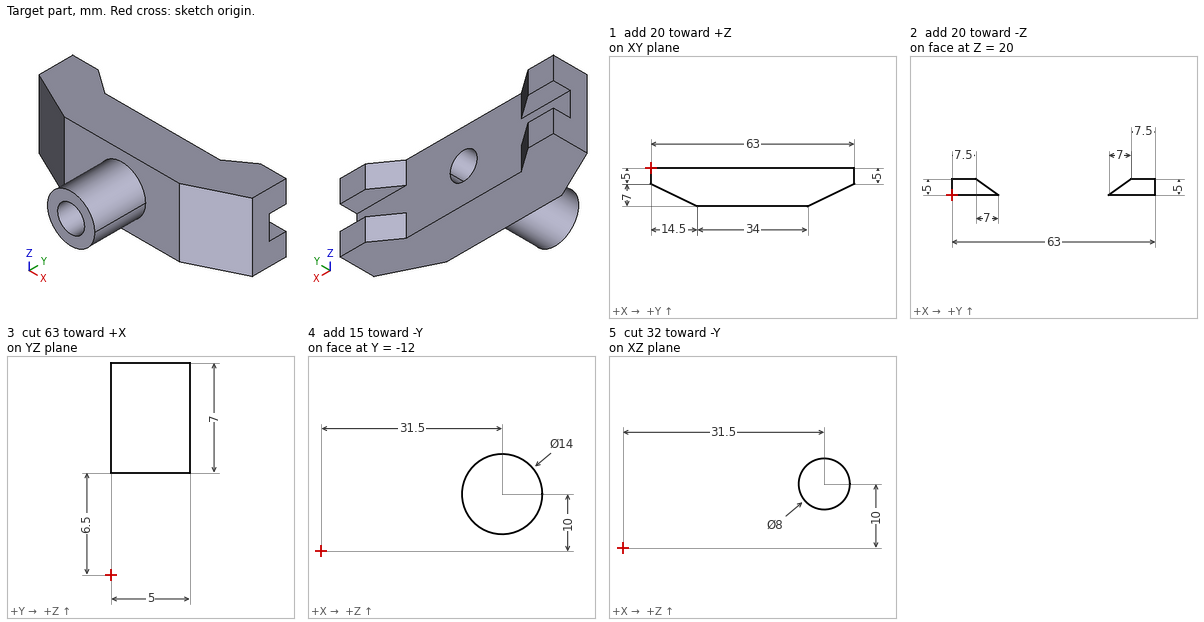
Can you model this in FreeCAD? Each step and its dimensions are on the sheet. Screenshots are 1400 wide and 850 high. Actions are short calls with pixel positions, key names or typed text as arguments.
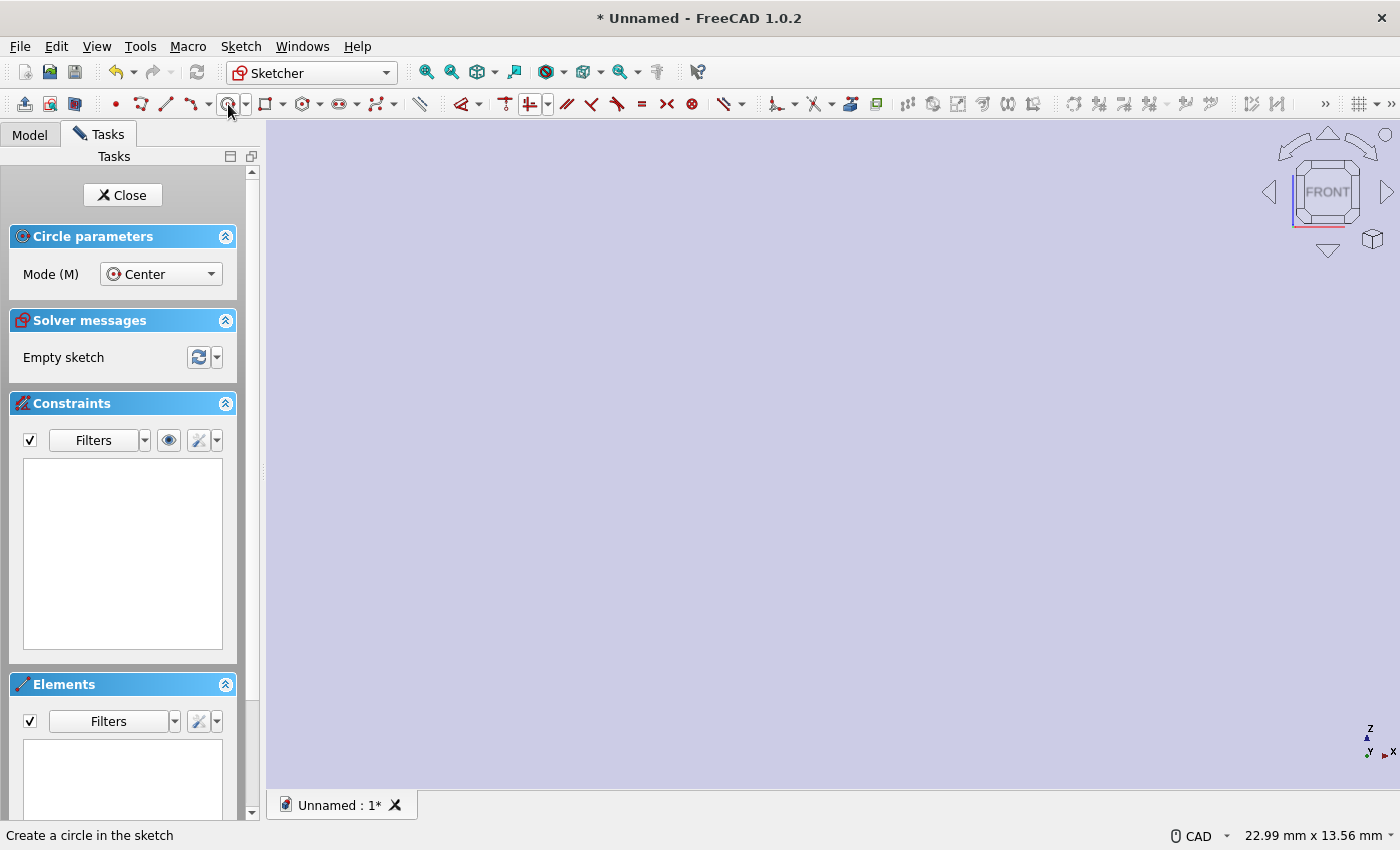
click(764, 454)
move(904, 314)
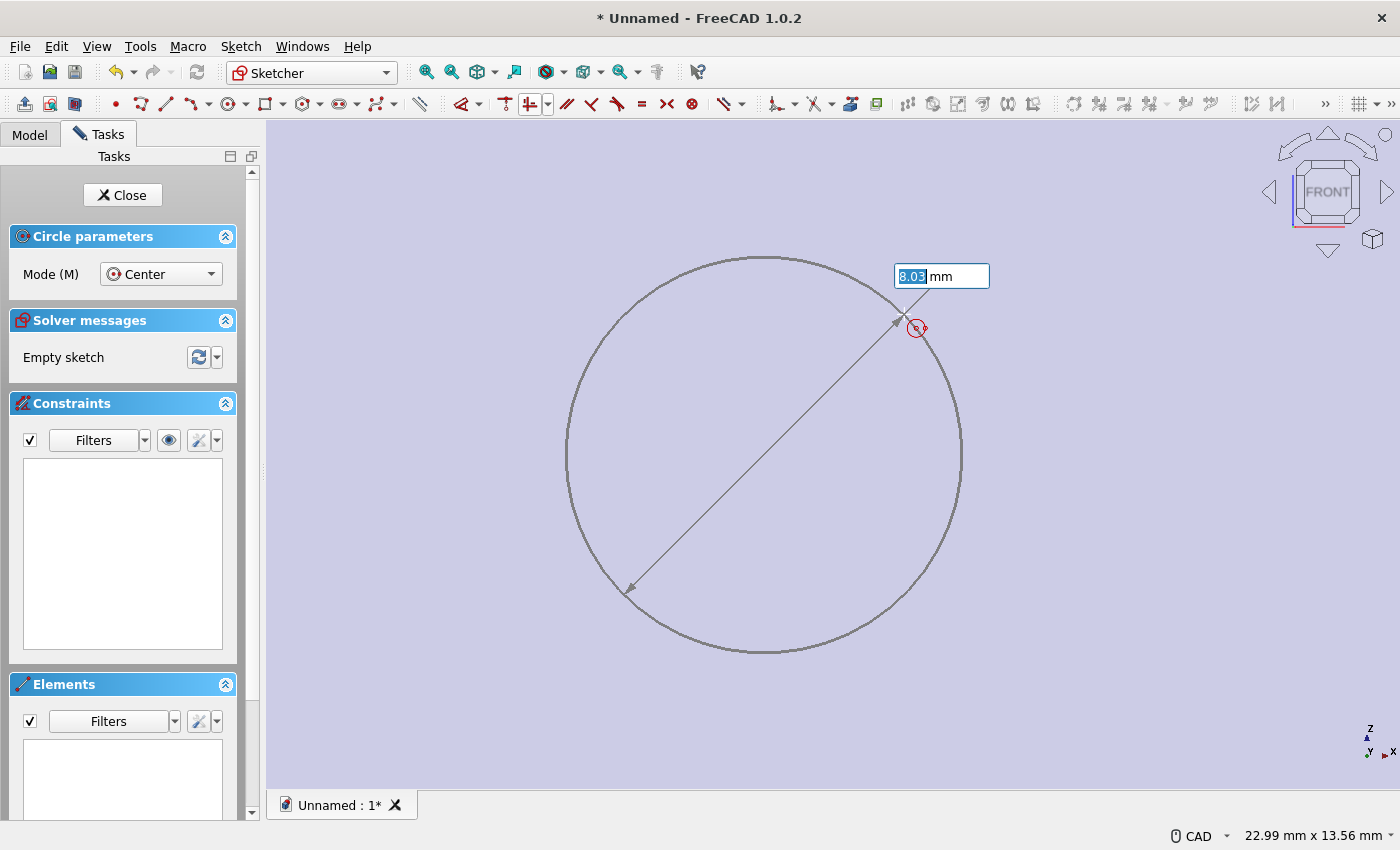
text(8)
key(Return)
key(Escape)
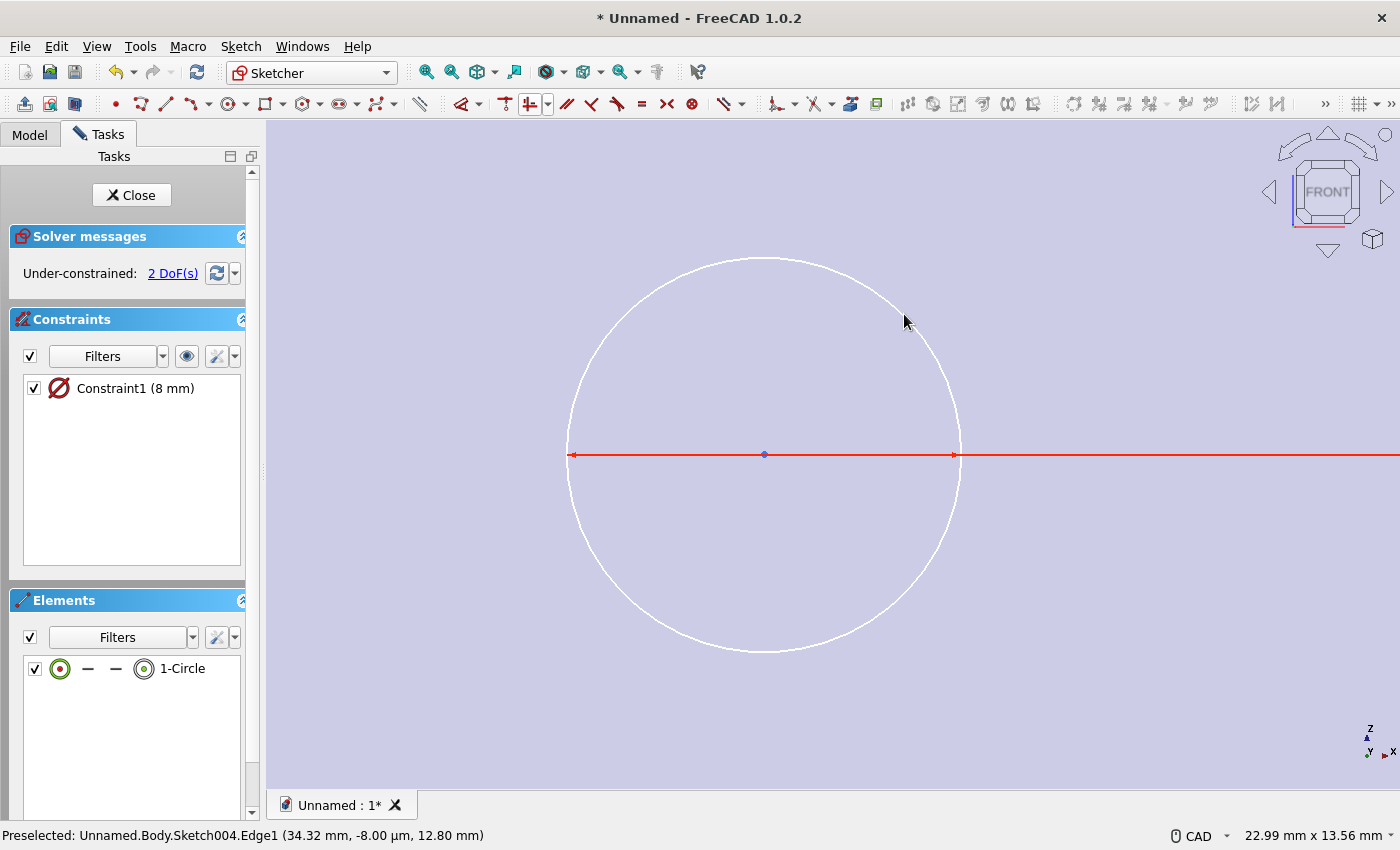
click(460, 104)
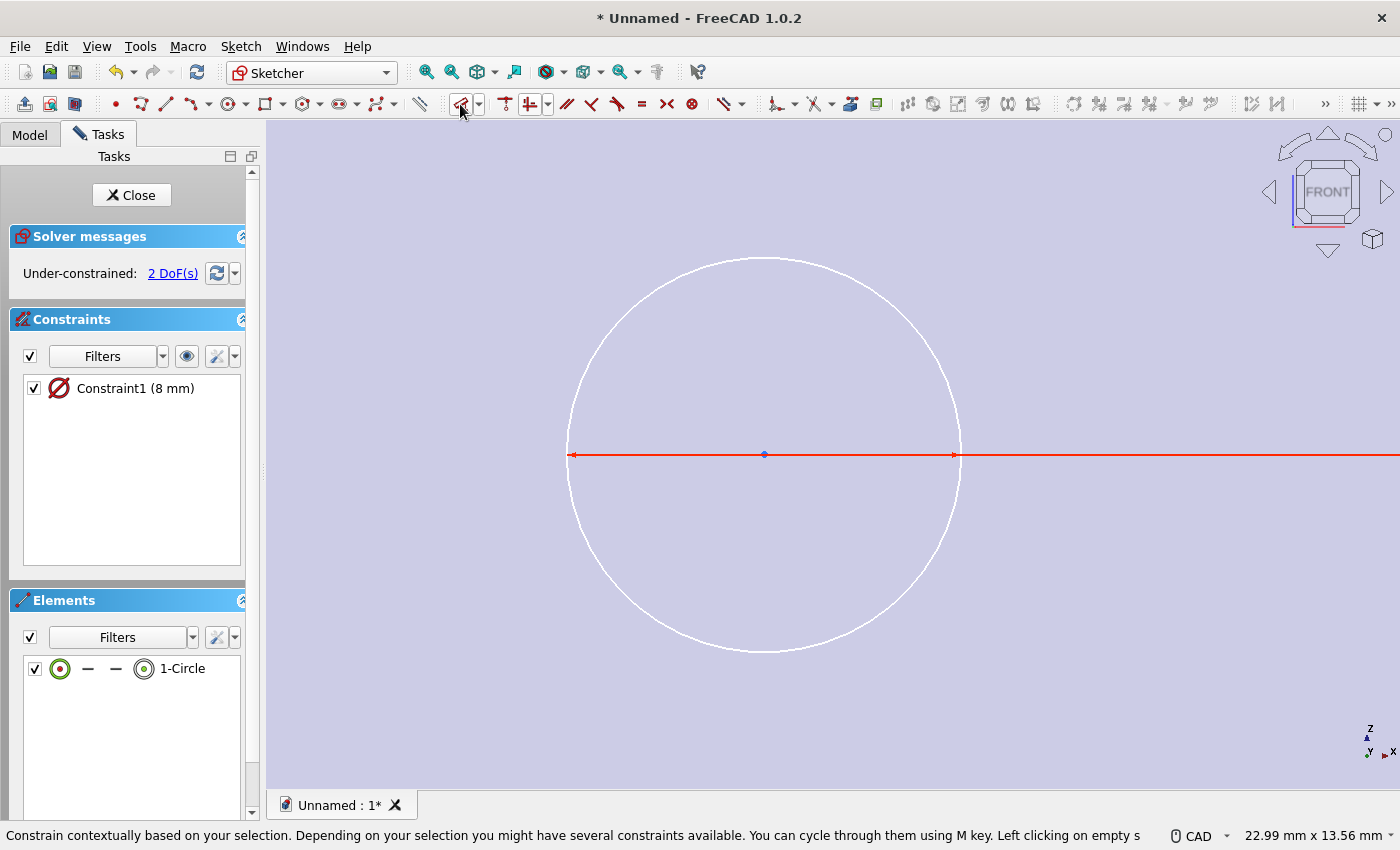
click(764, 455)
click(798, 608)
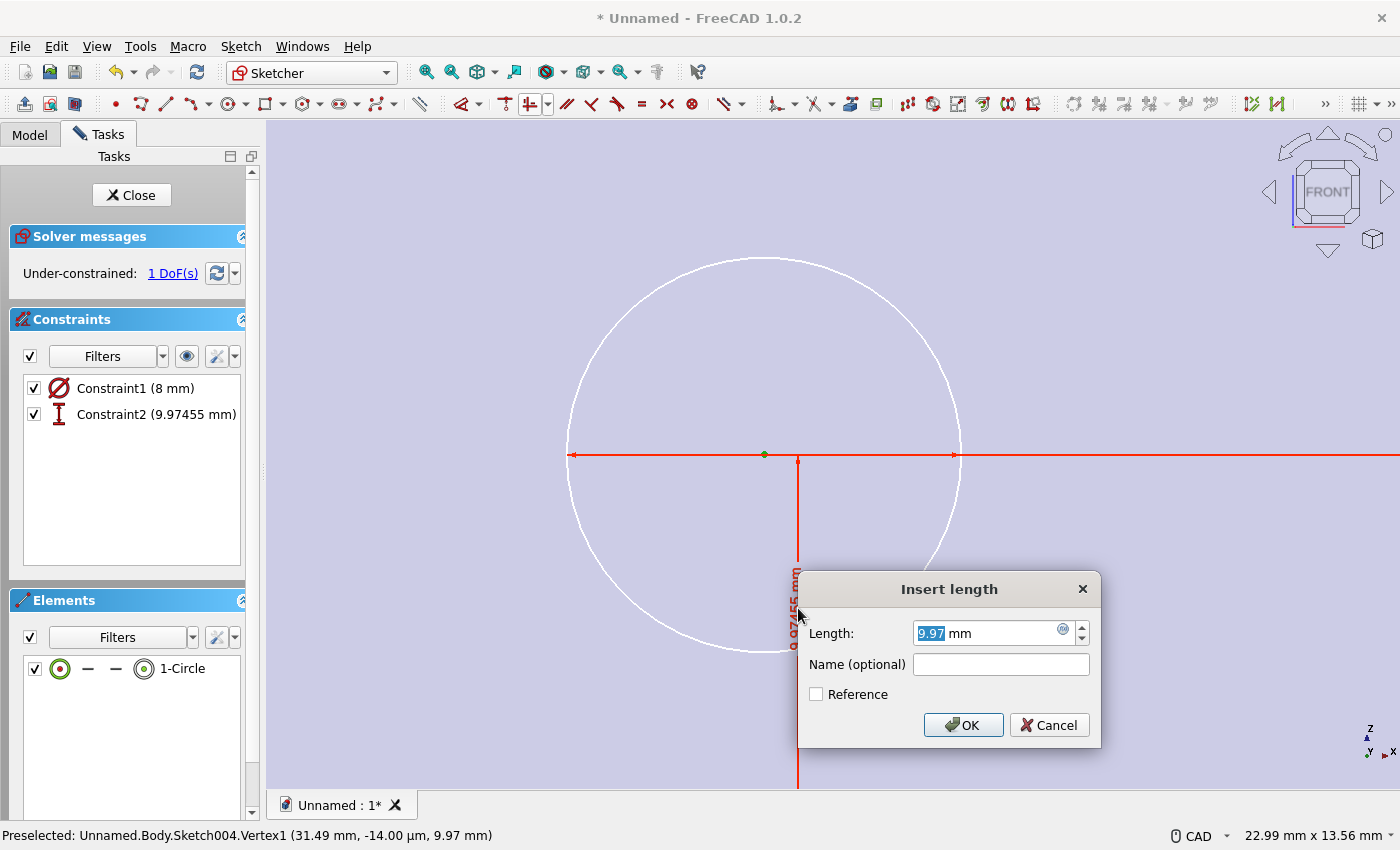
text(10)
key(Return)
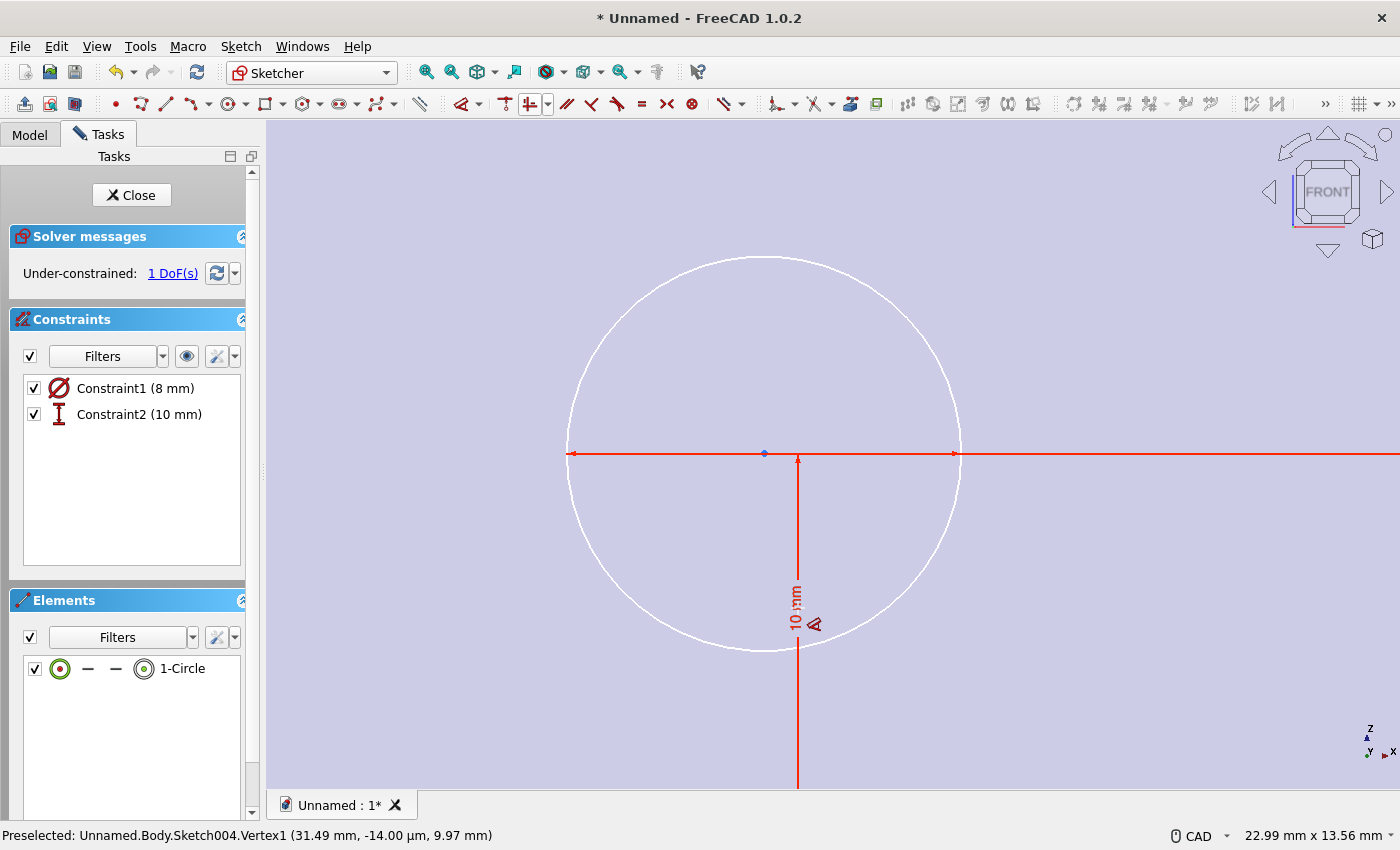
click(764, 454)
click(529, 420)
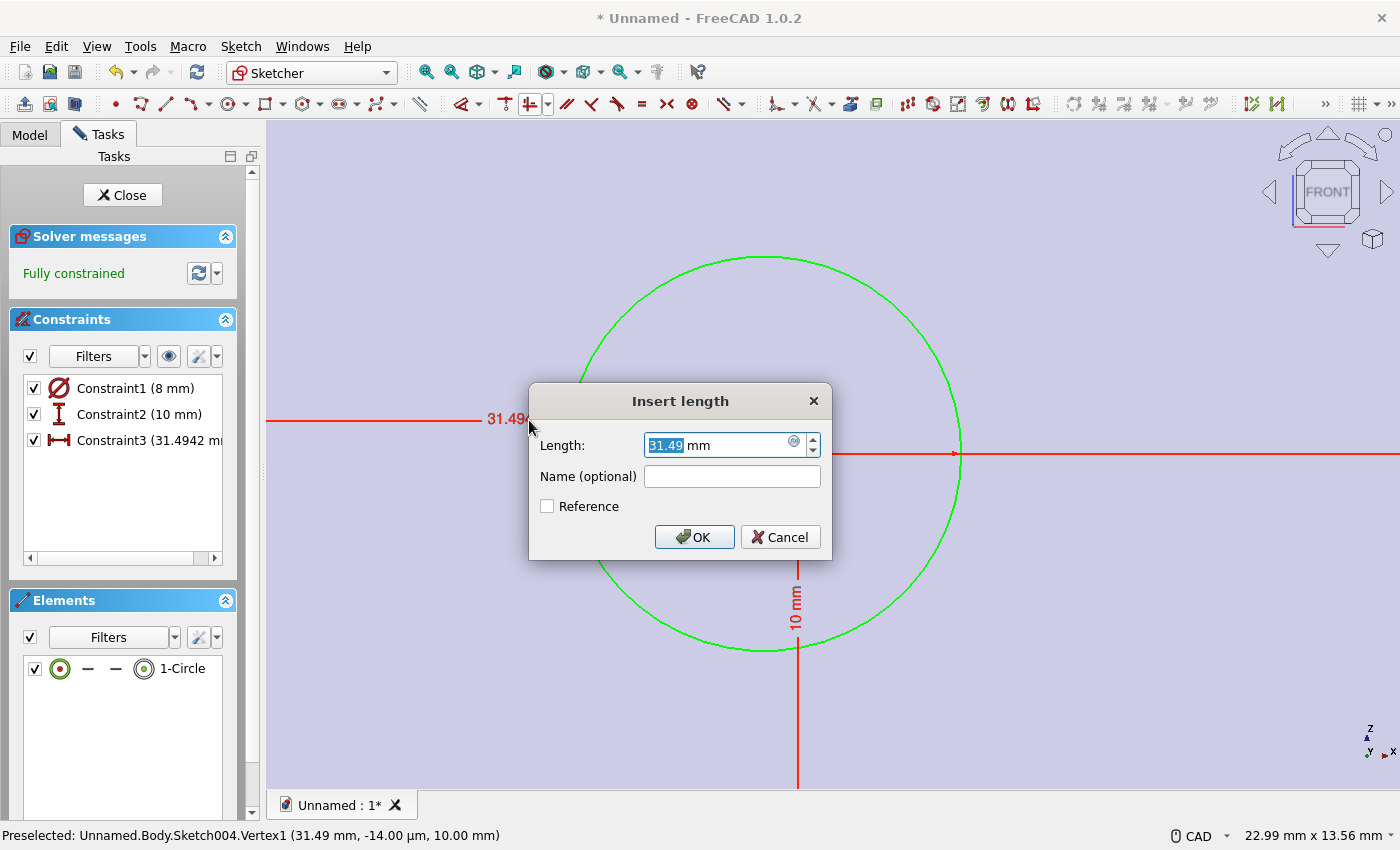
text(31.5)
key(Return)
key(Escape)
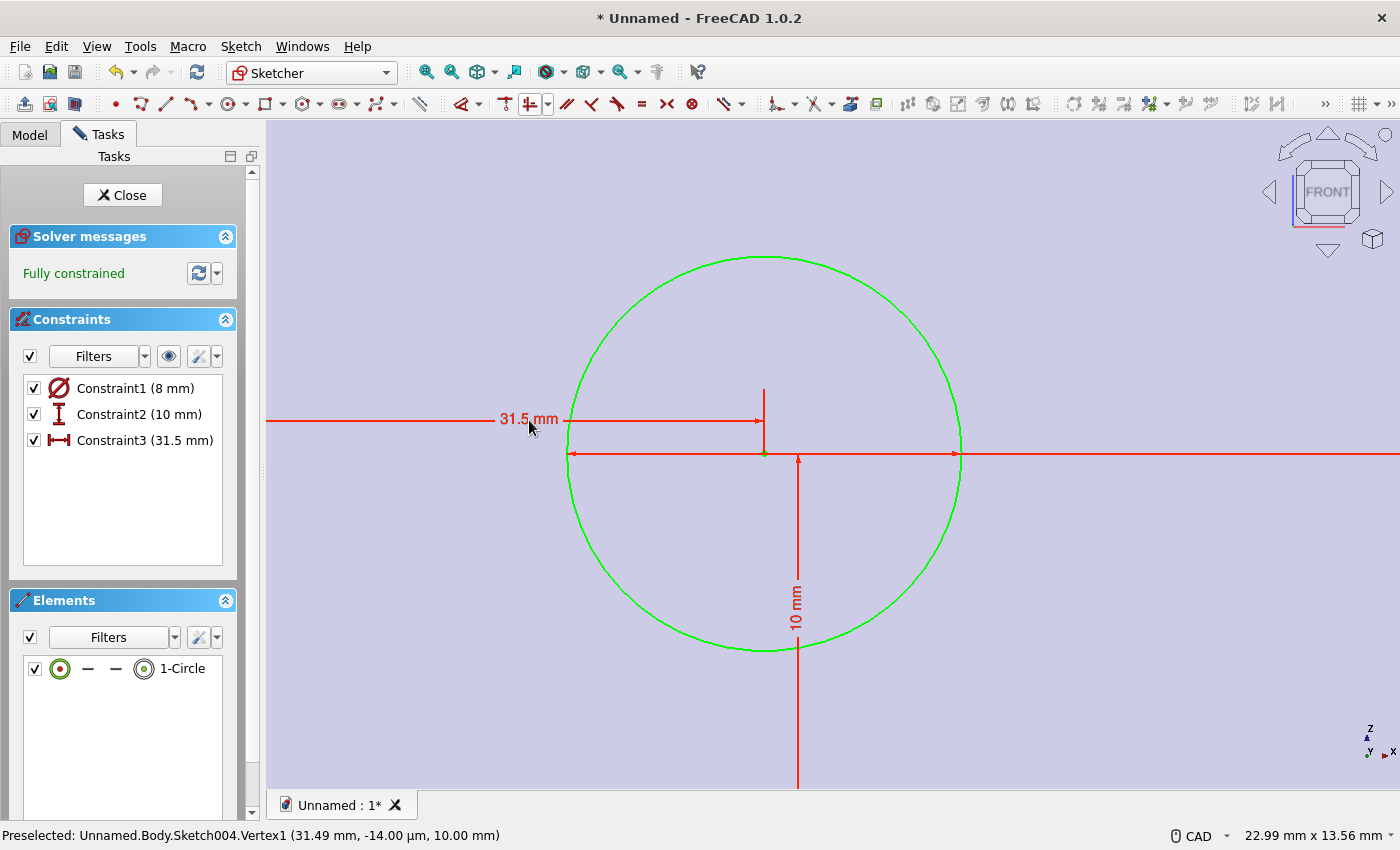
click(123, 195)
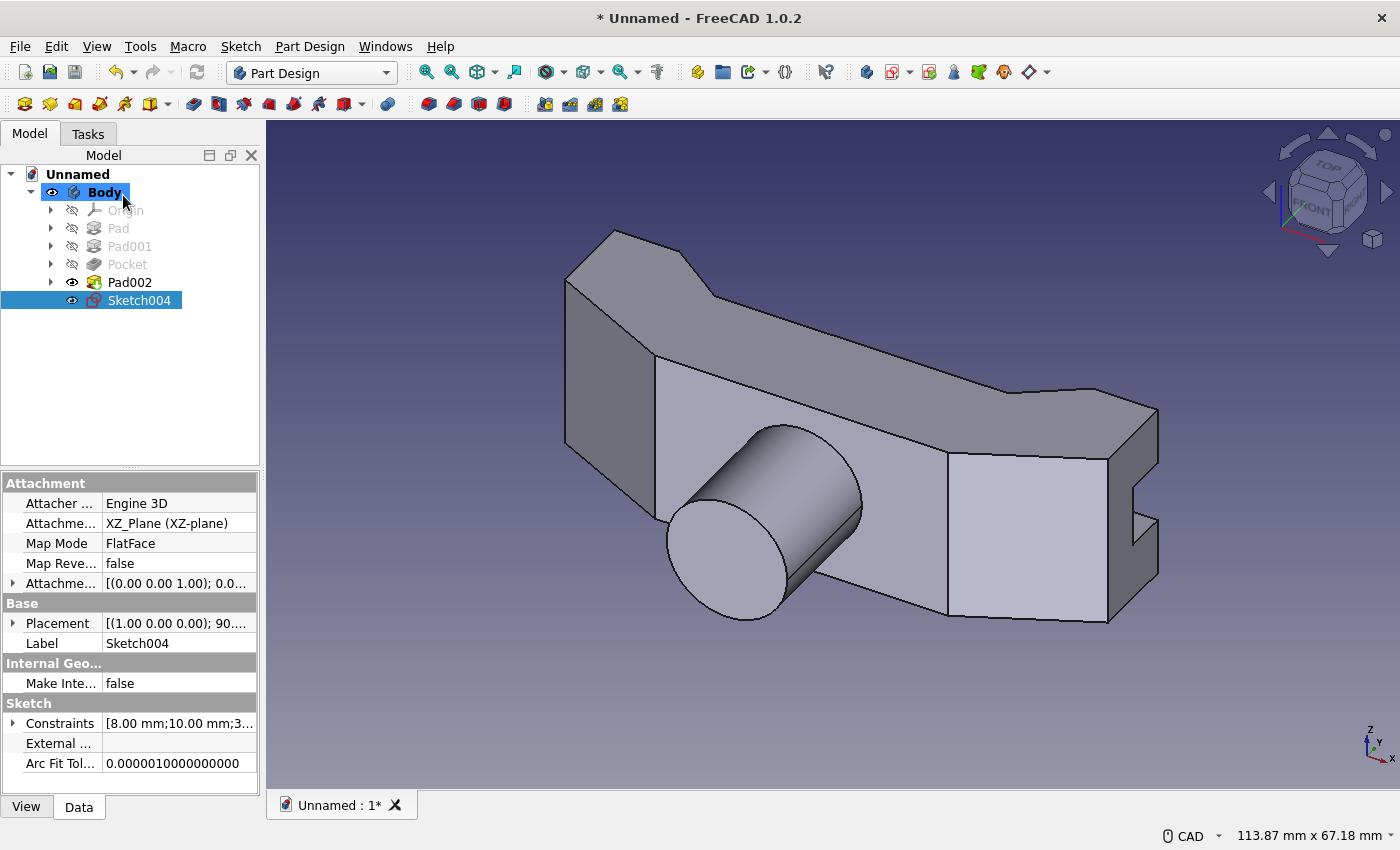
click(194, 104)